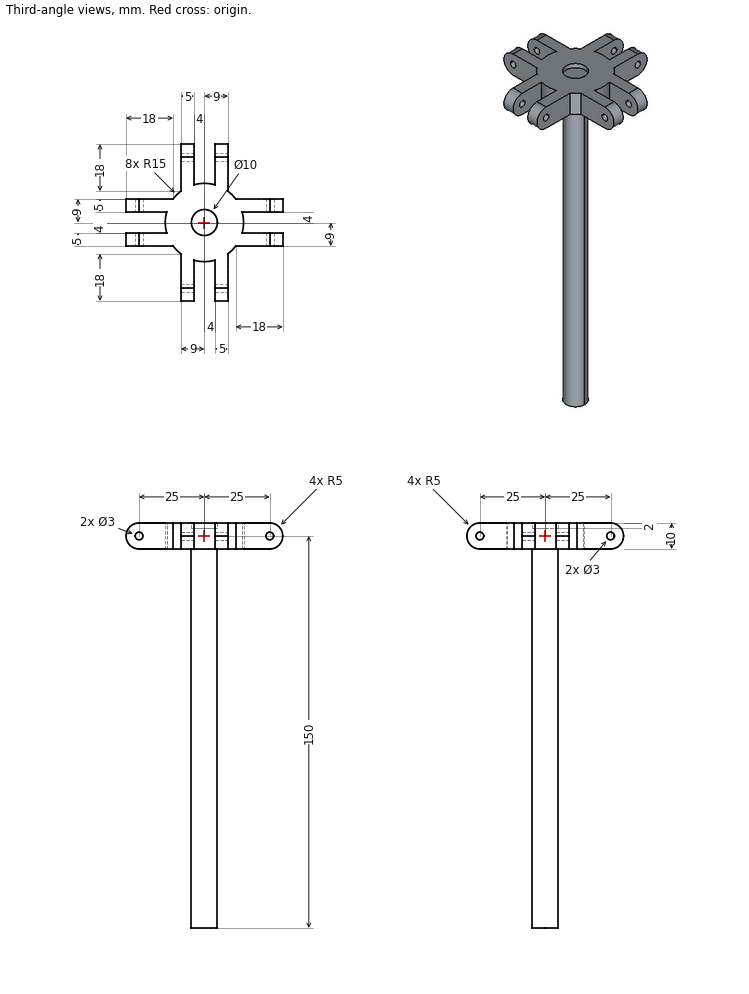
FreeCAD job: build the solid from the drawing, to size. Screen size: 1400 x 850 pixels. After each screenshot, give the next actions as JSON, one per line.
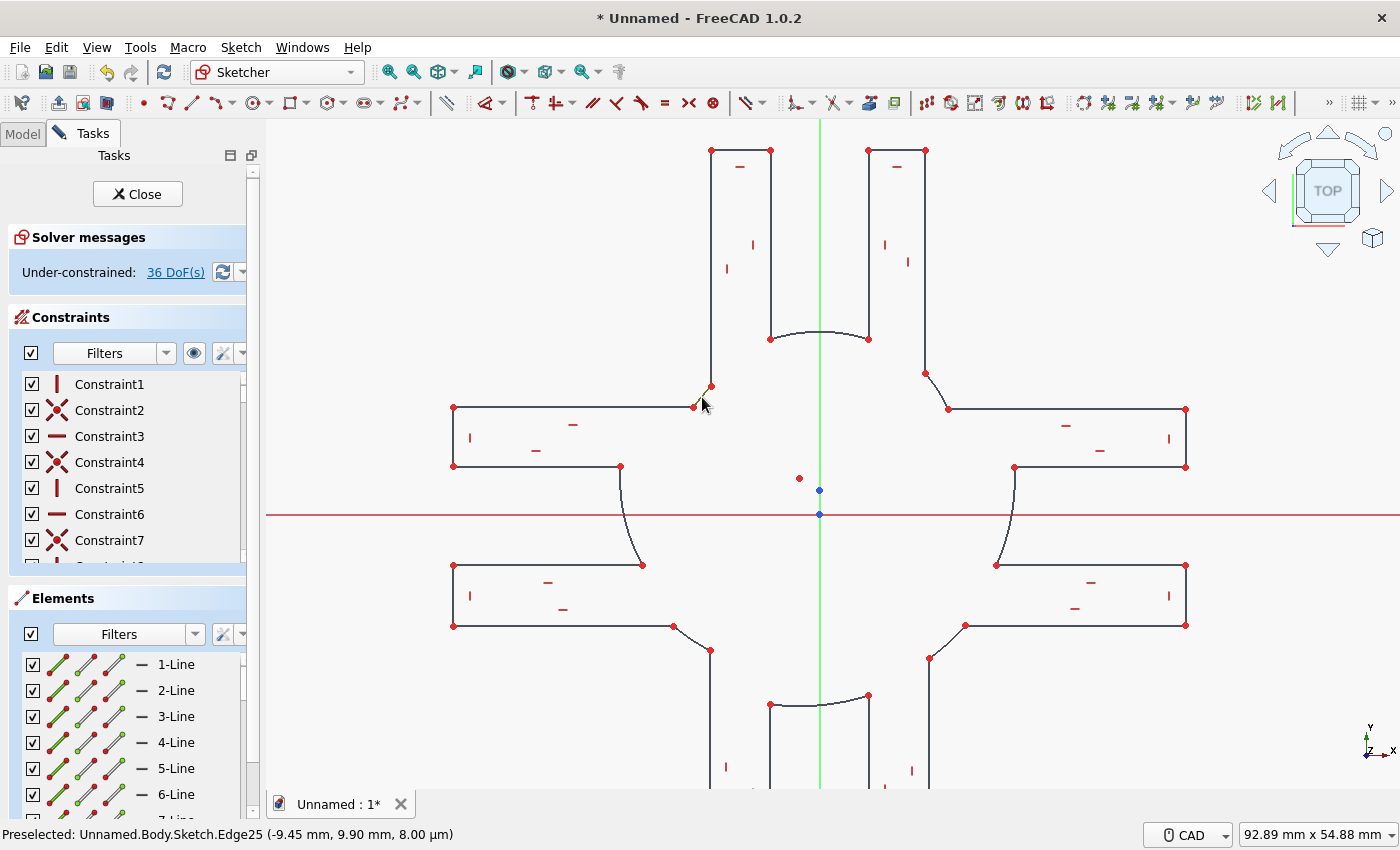
{"action": "left_click", "coordinate": [840, 333]}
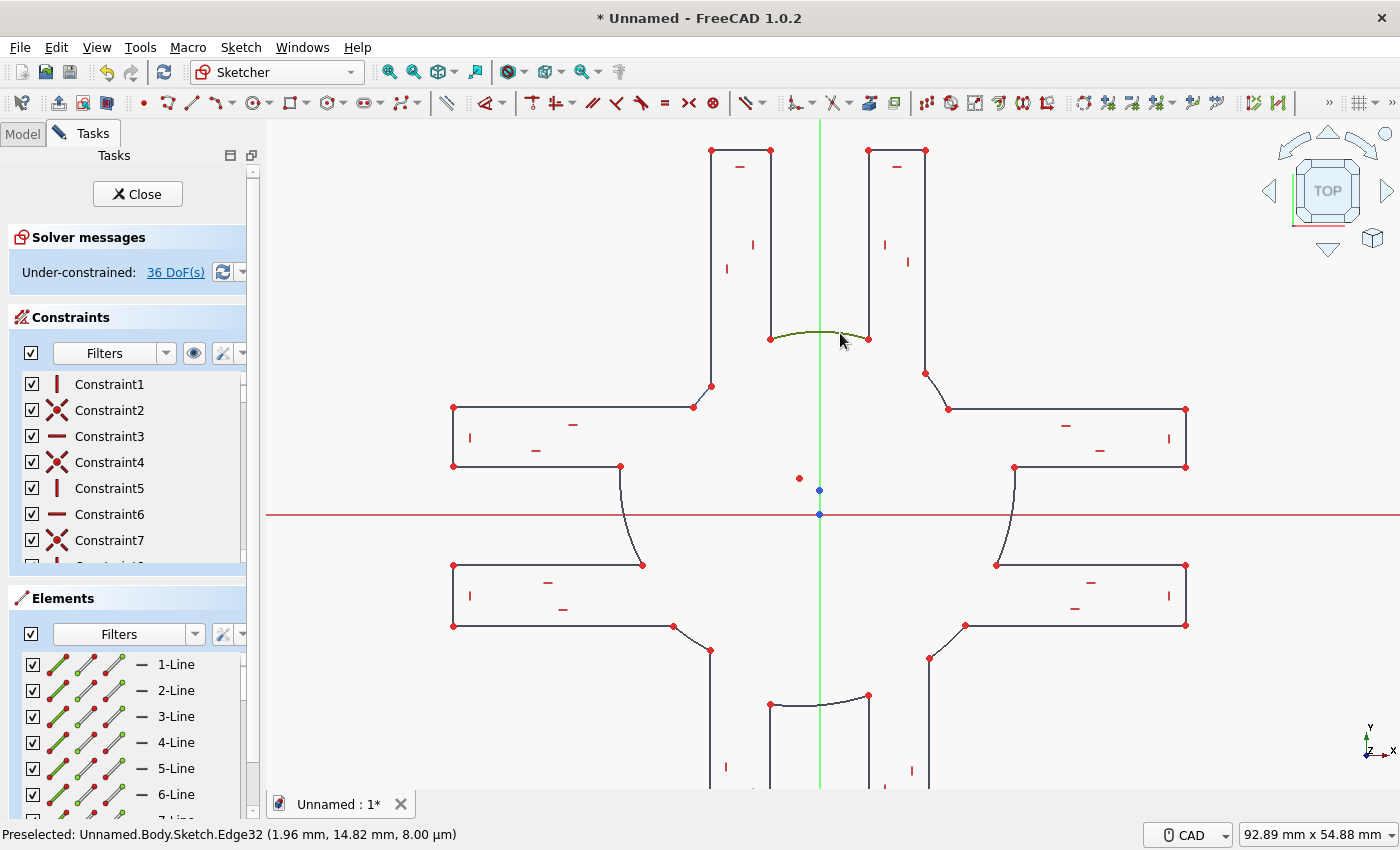
{"action": "key", "text": "c"}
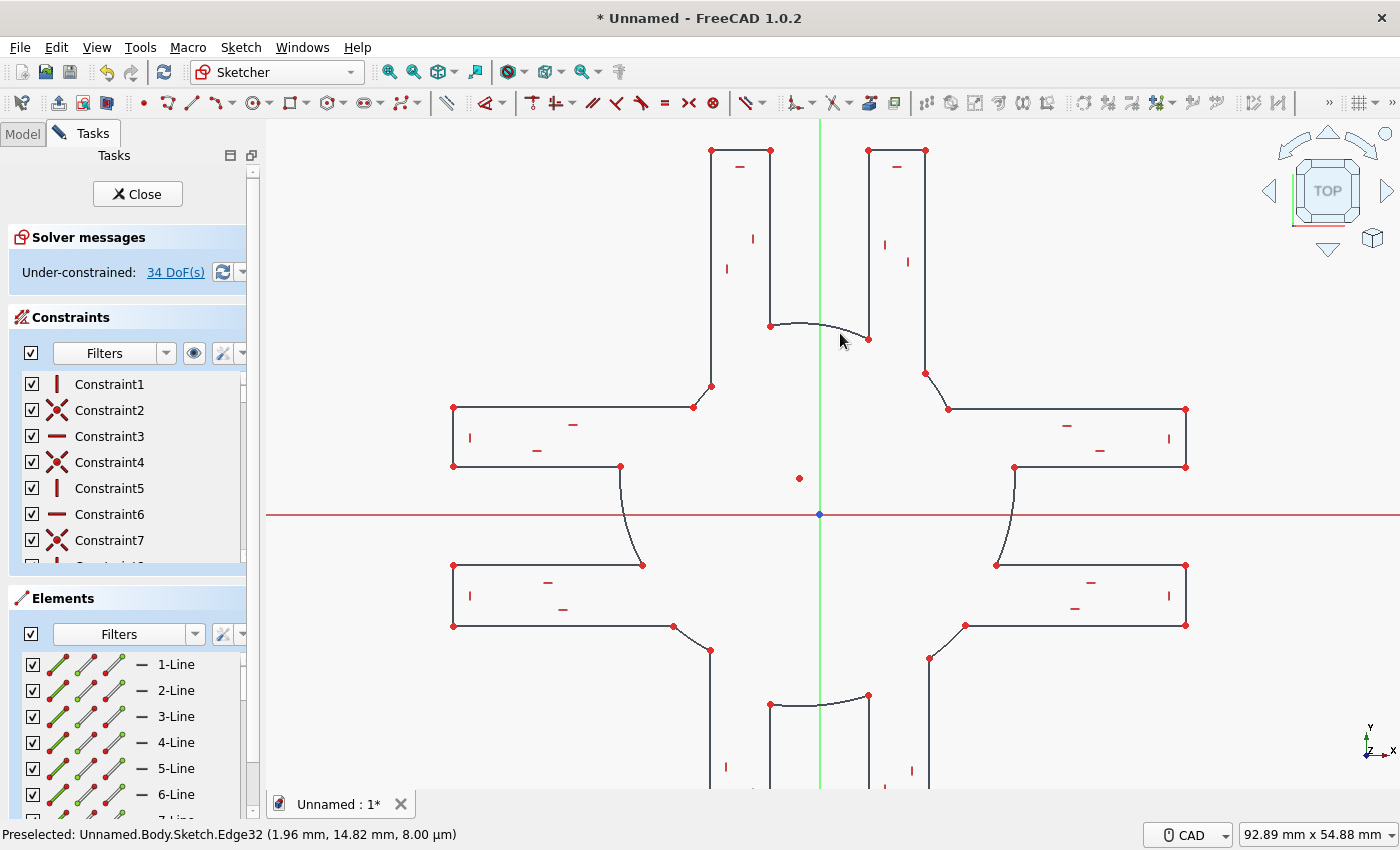
{"action": "left_click_drag", "start_coordinate": [790, 468], "coordinate": [830, 525]}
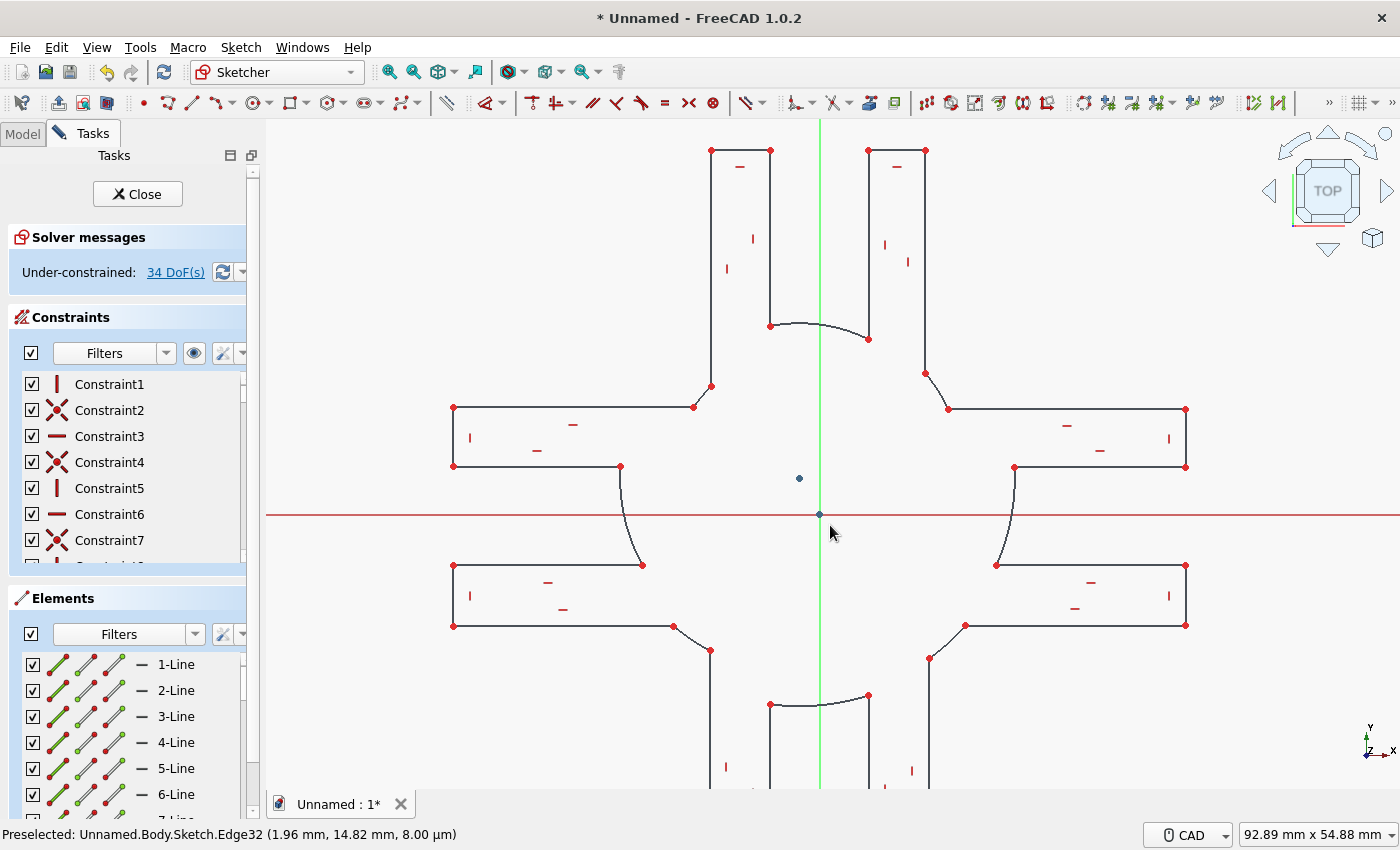
{"action": "left_click", "coordinate": [532, 104]}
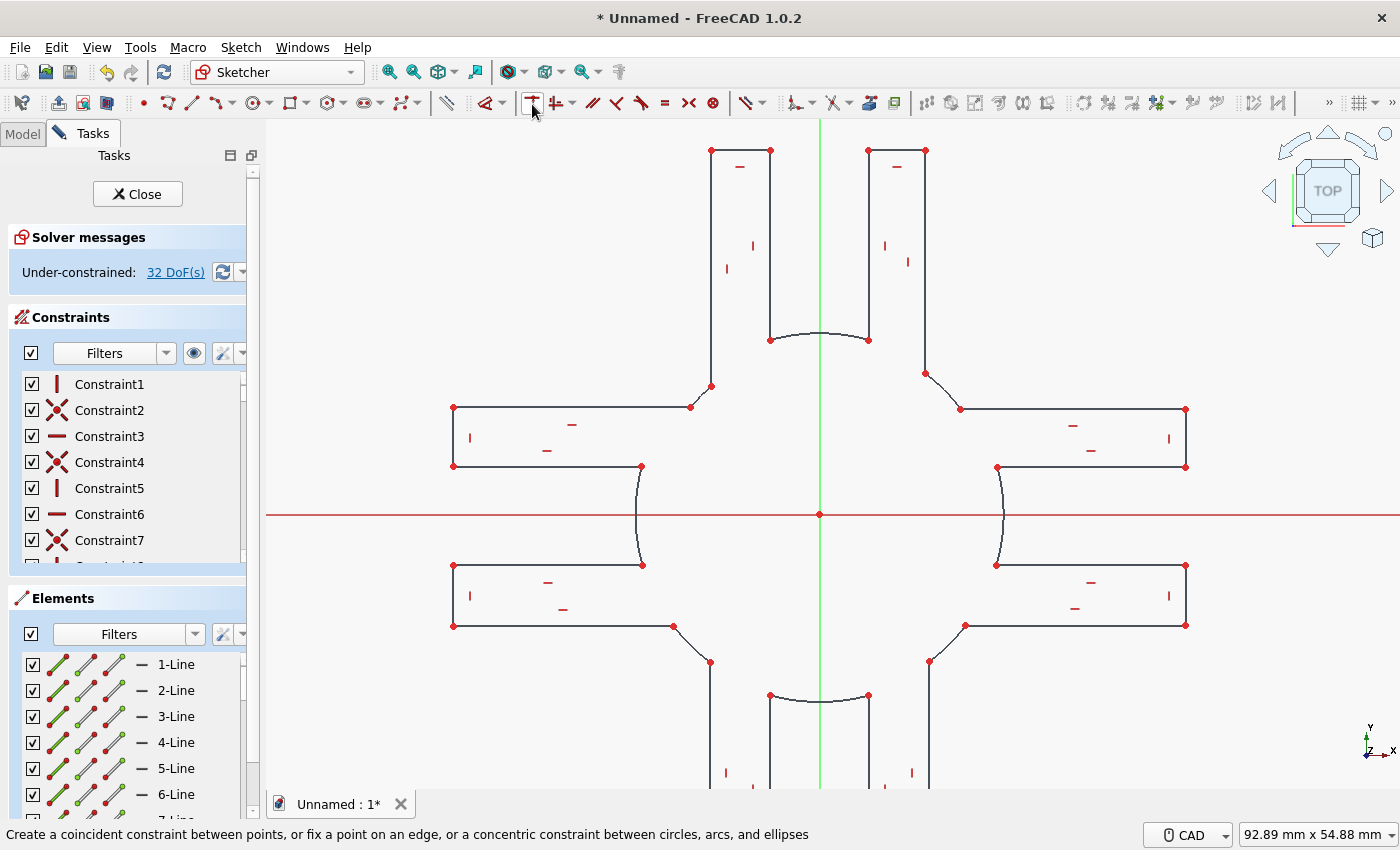
{"action": "left_click", "coordinate": [700, 397]}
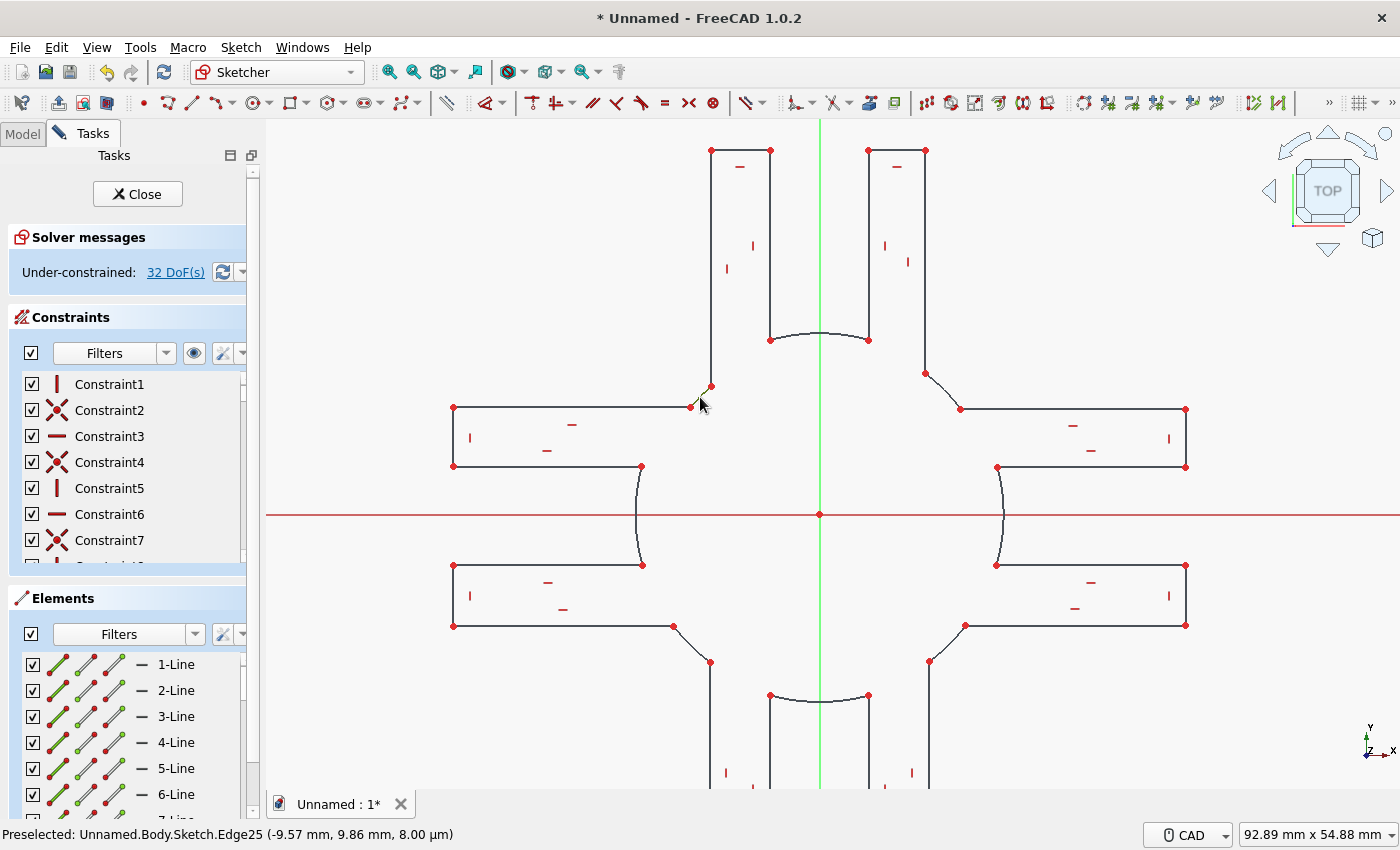
{"action": "left_click", "coordinate": [636, 496]}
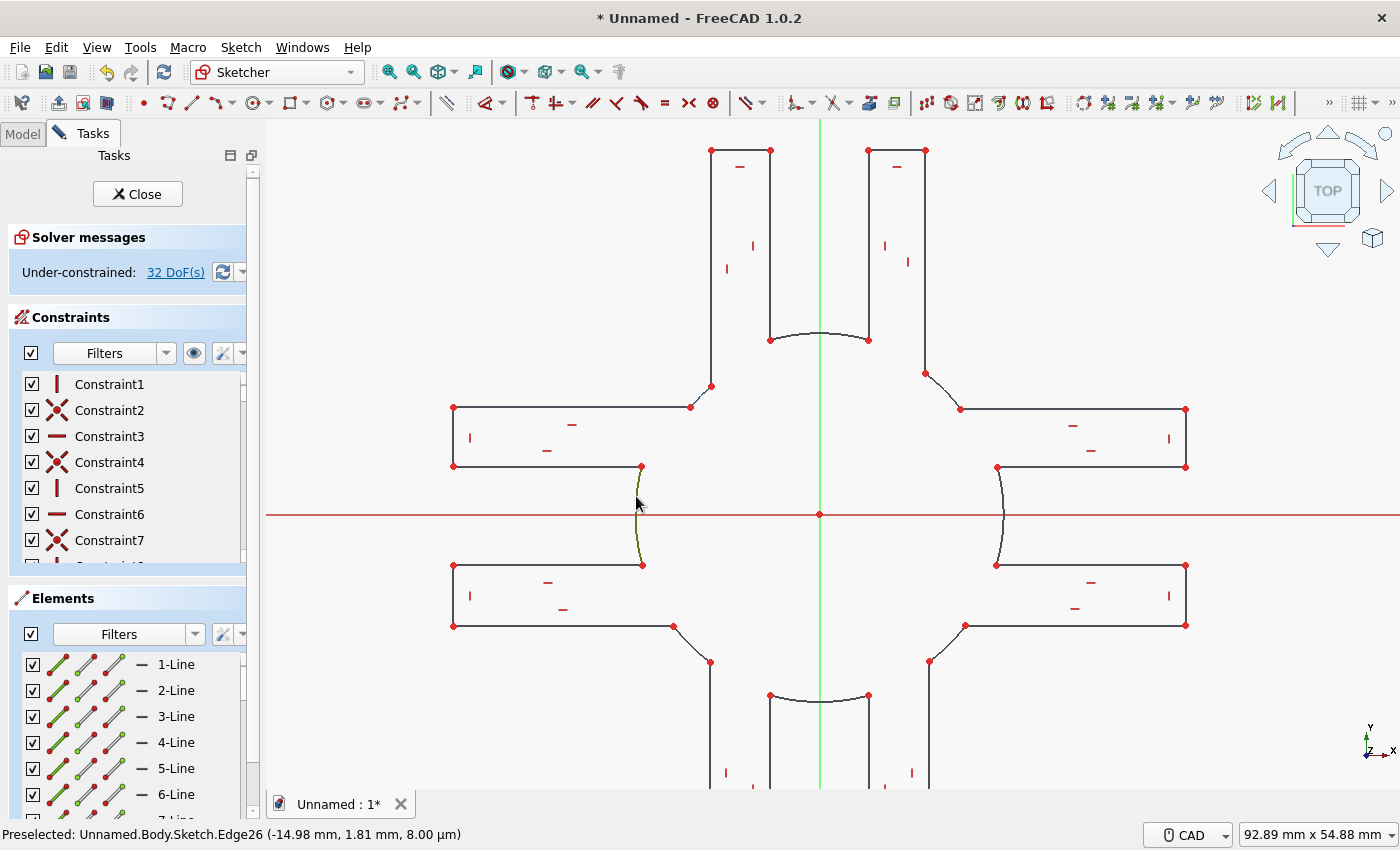
{"action": "left_click", "coordinate": [683, 638]}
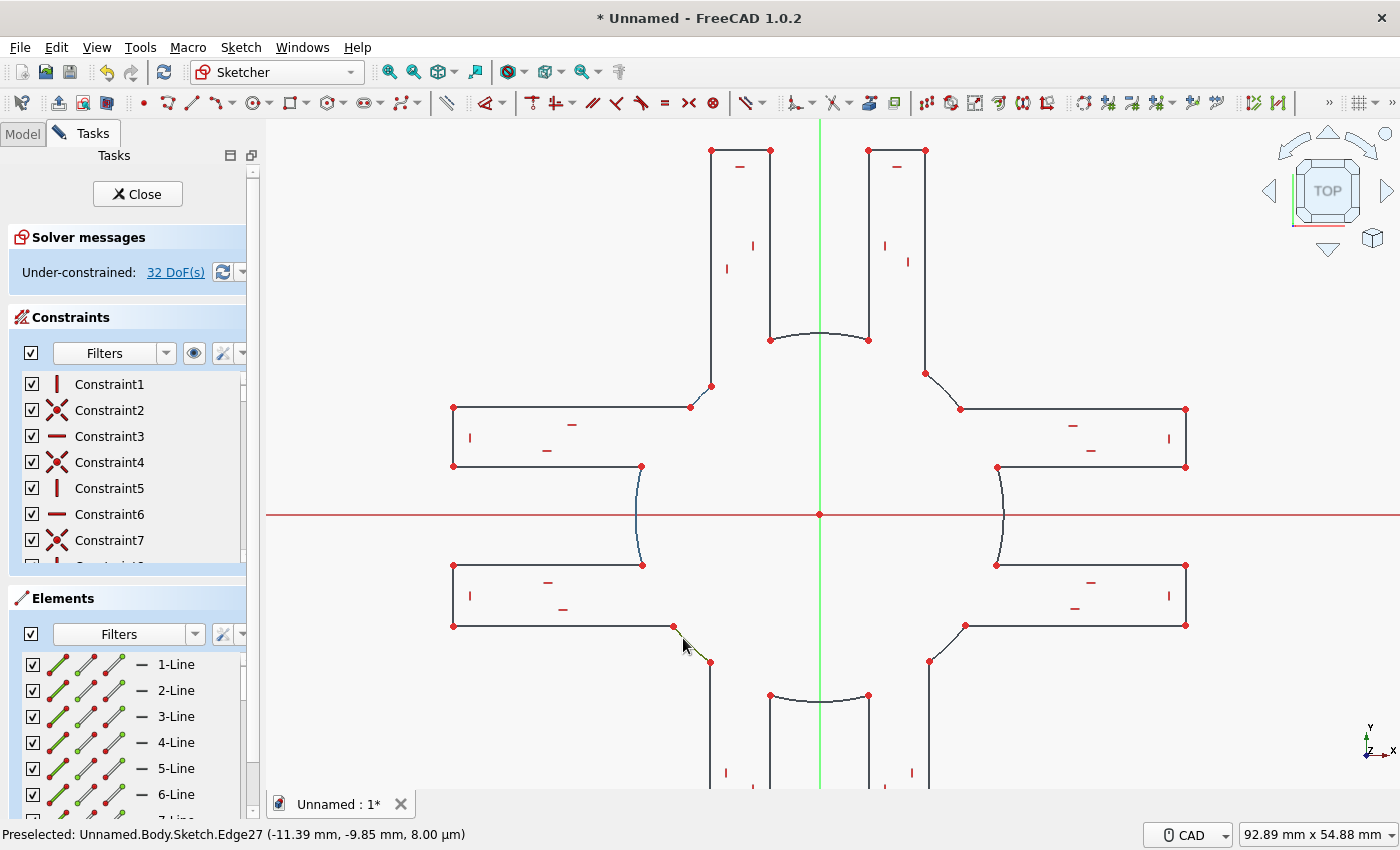
{"action": "left_click", "coordinate": [800, 701]}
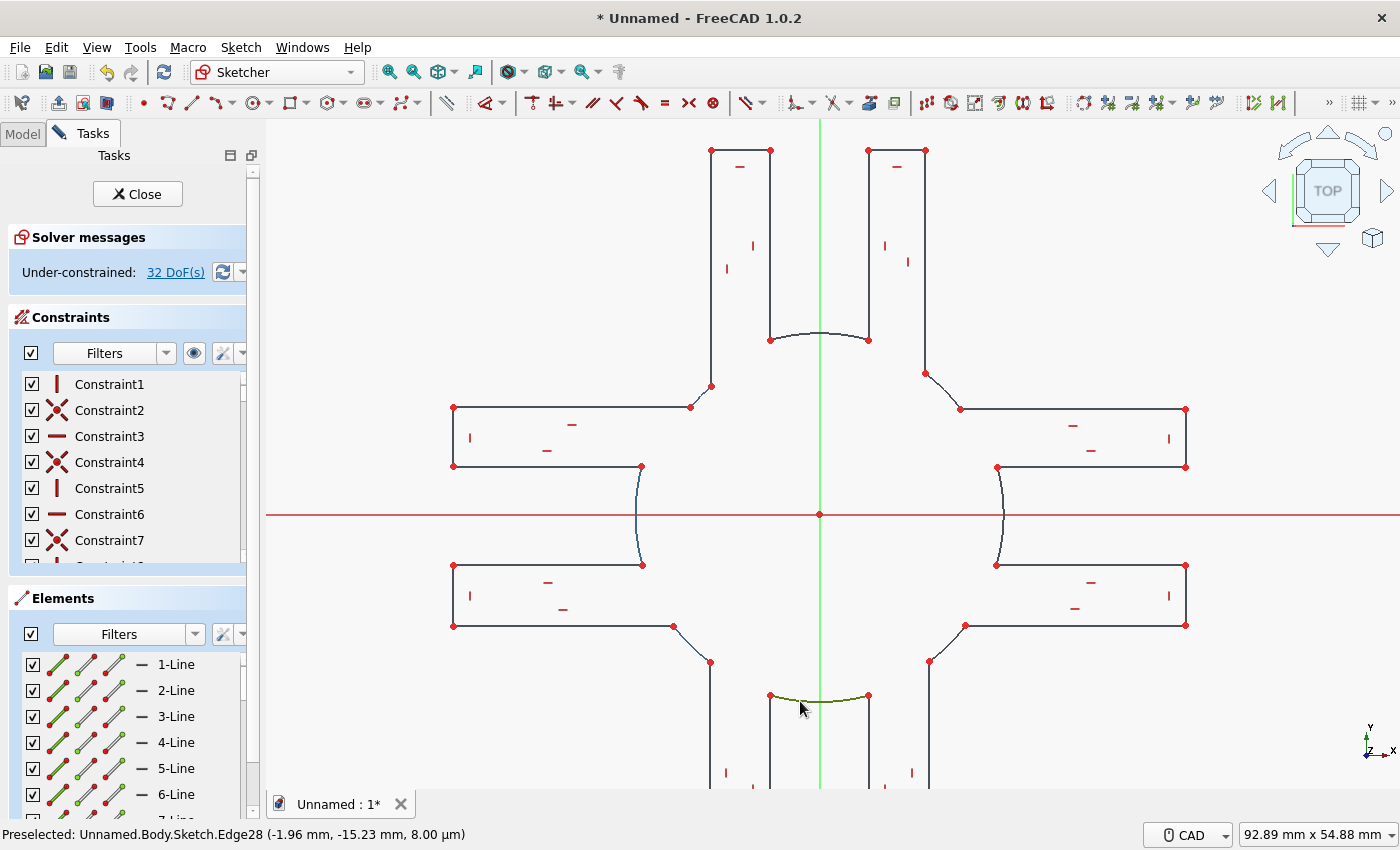
{"action": "left_click", "coordinate": [941, 652]}